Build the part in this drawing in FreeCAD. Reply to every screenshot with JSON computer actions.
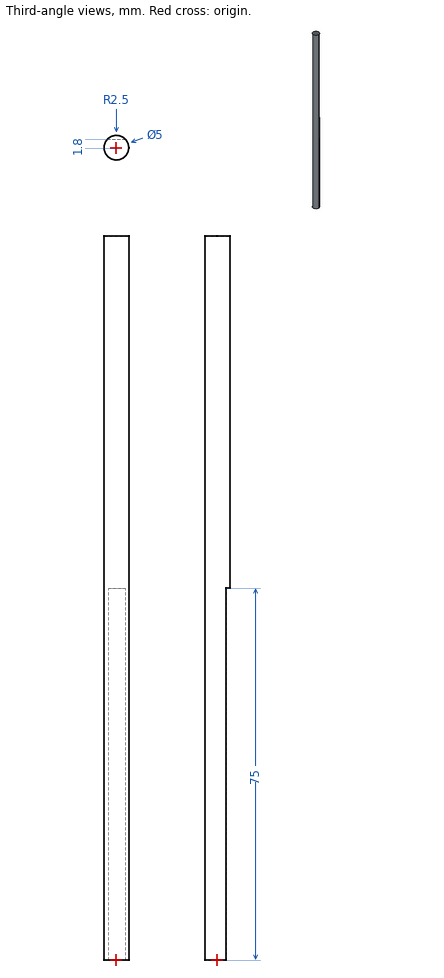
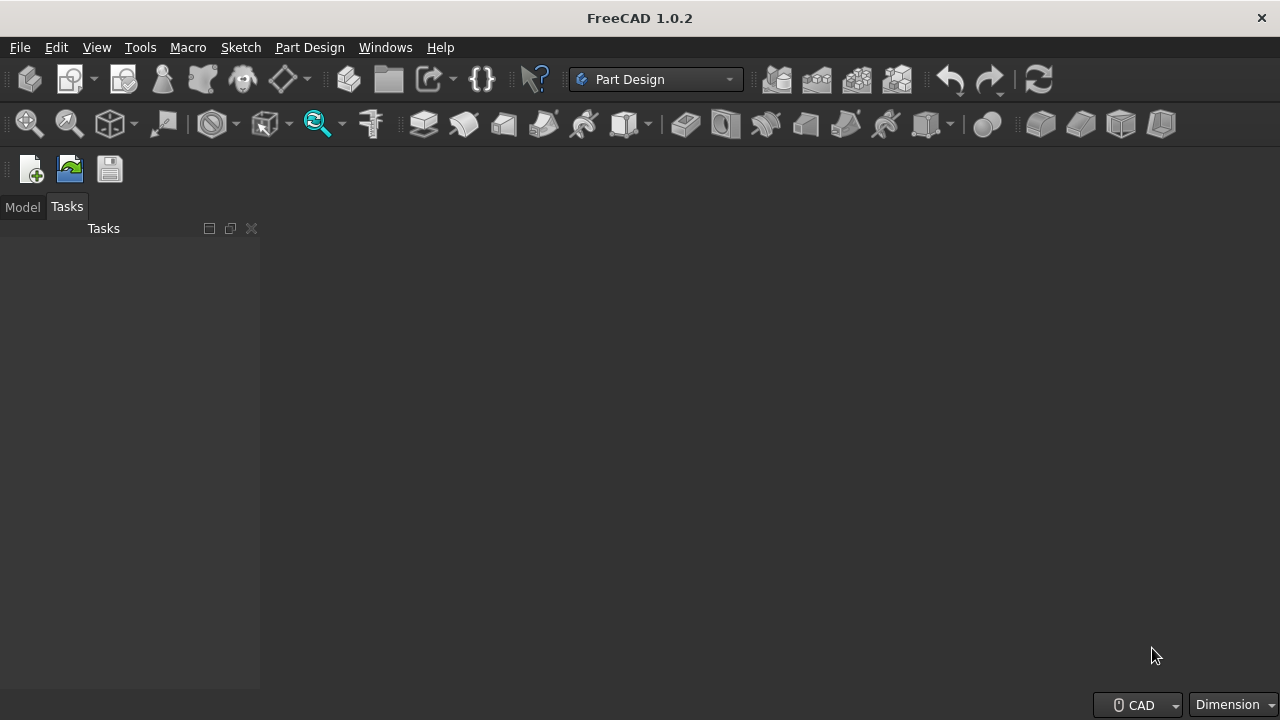
{"action": "key", "text": "ctrl+n"}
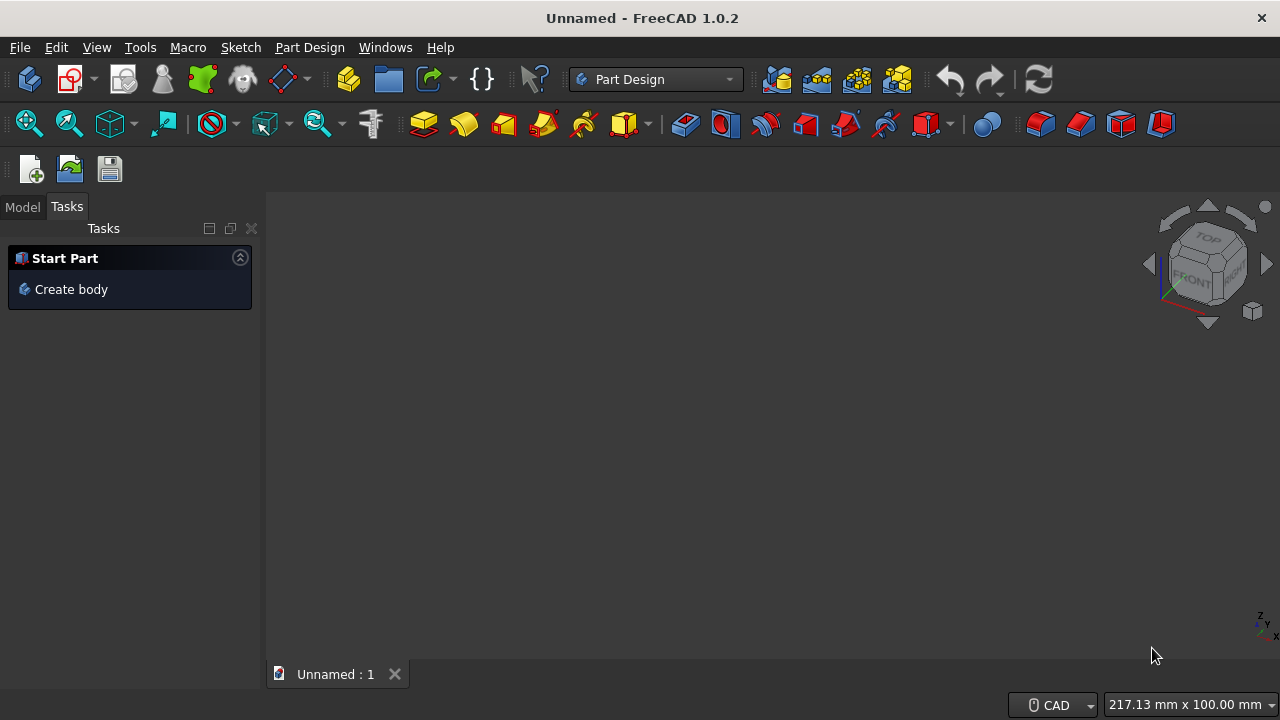
{"action": "left_click", "coordinate": [70, 80]}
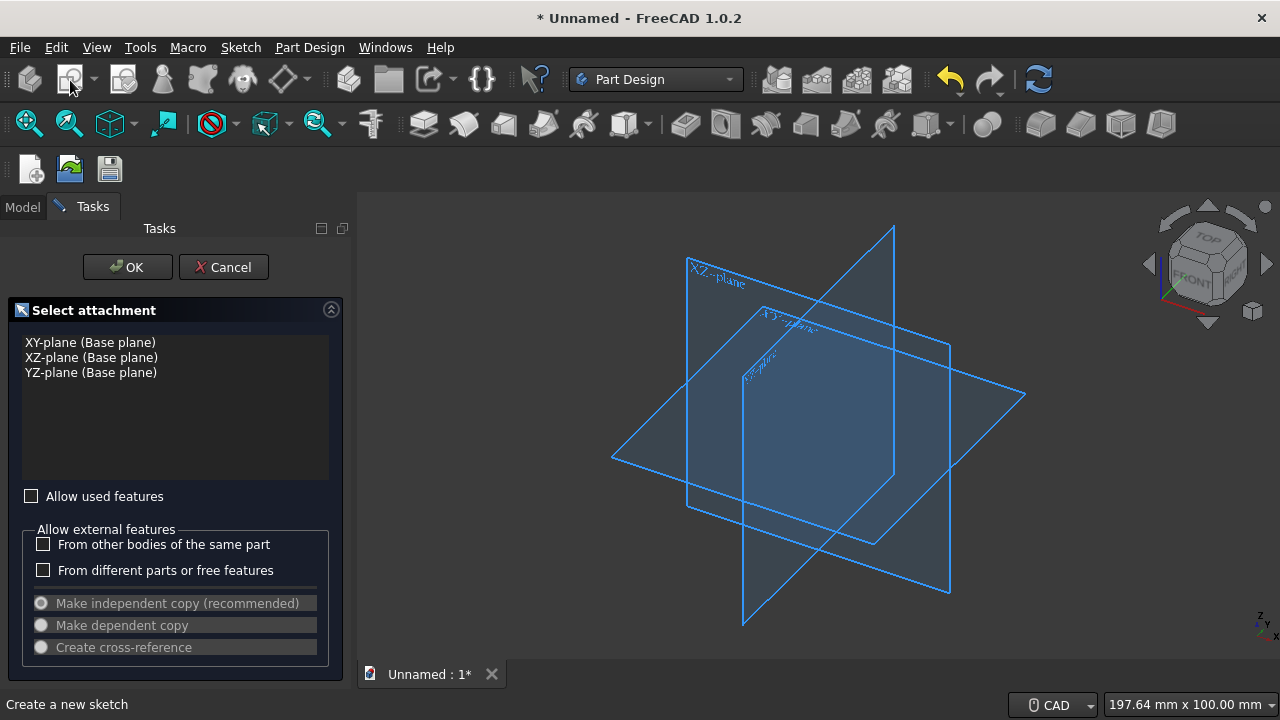
{"action": "left_click", "coordinate": [82, 342]}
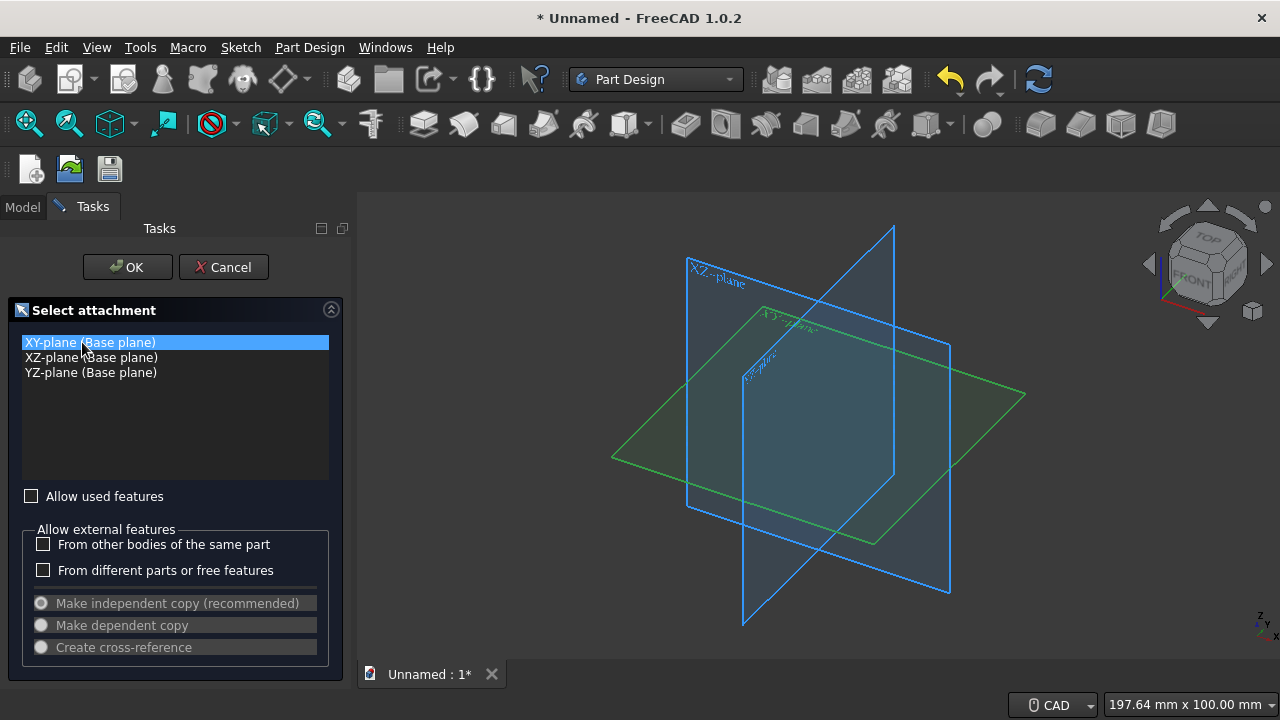
{"action": "left_click", "coordinate": [128, 267]}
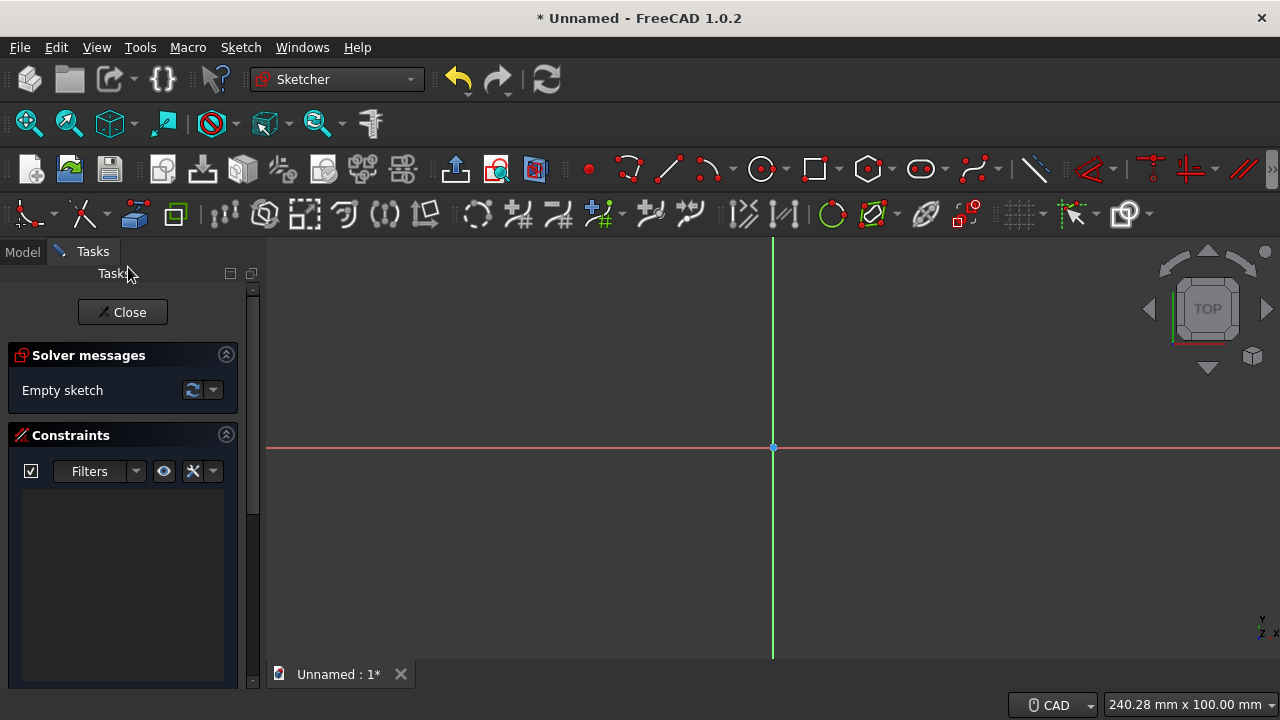
{"action": "scroll", "coordinate": [778, 448], "scroll_direction": "up", "scroll_amount": 13}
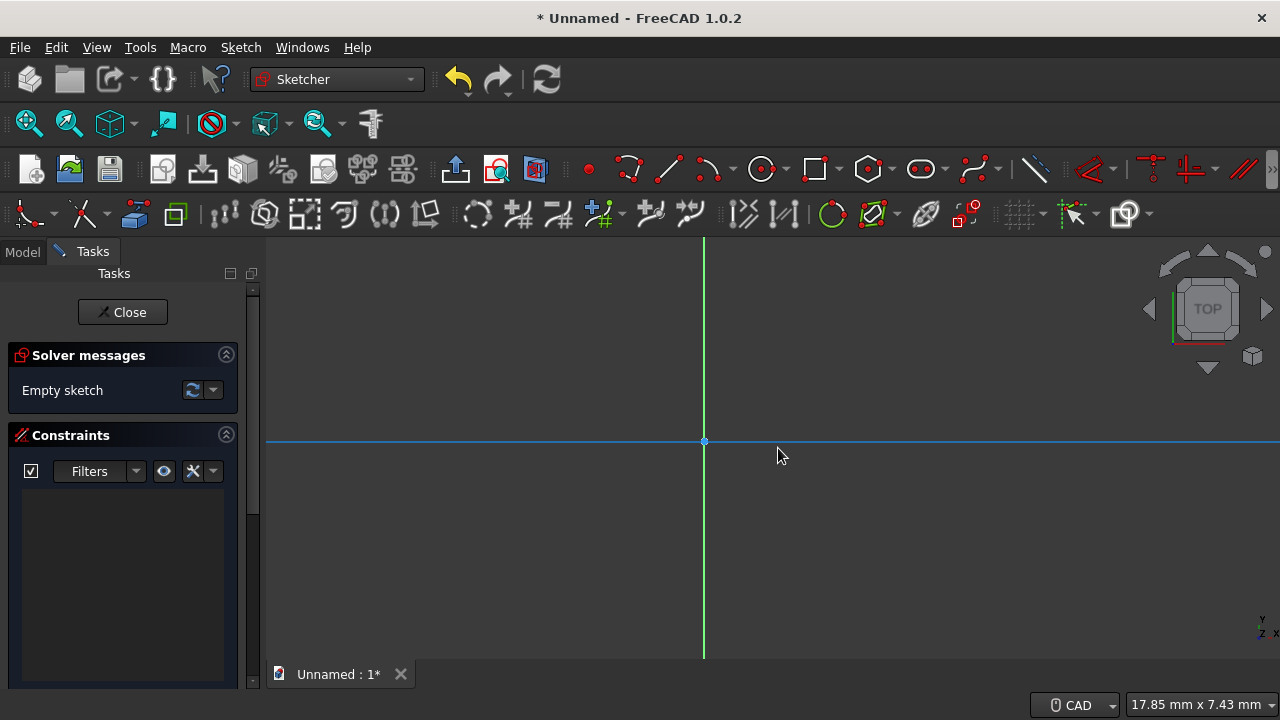
{"action": "key", "text": "g c"}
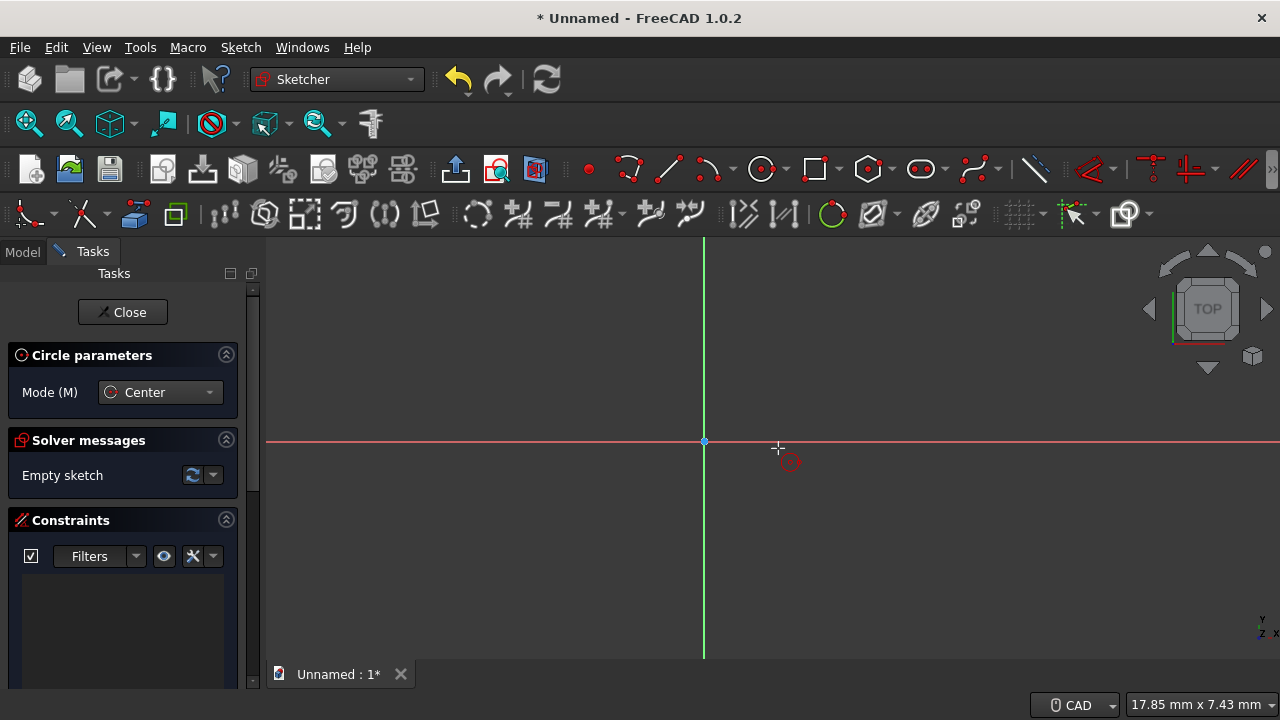
{"action": "left_click", "coordinate": [704, 442]}
{"action": "mouse_move", "coordinate": [805, 341]}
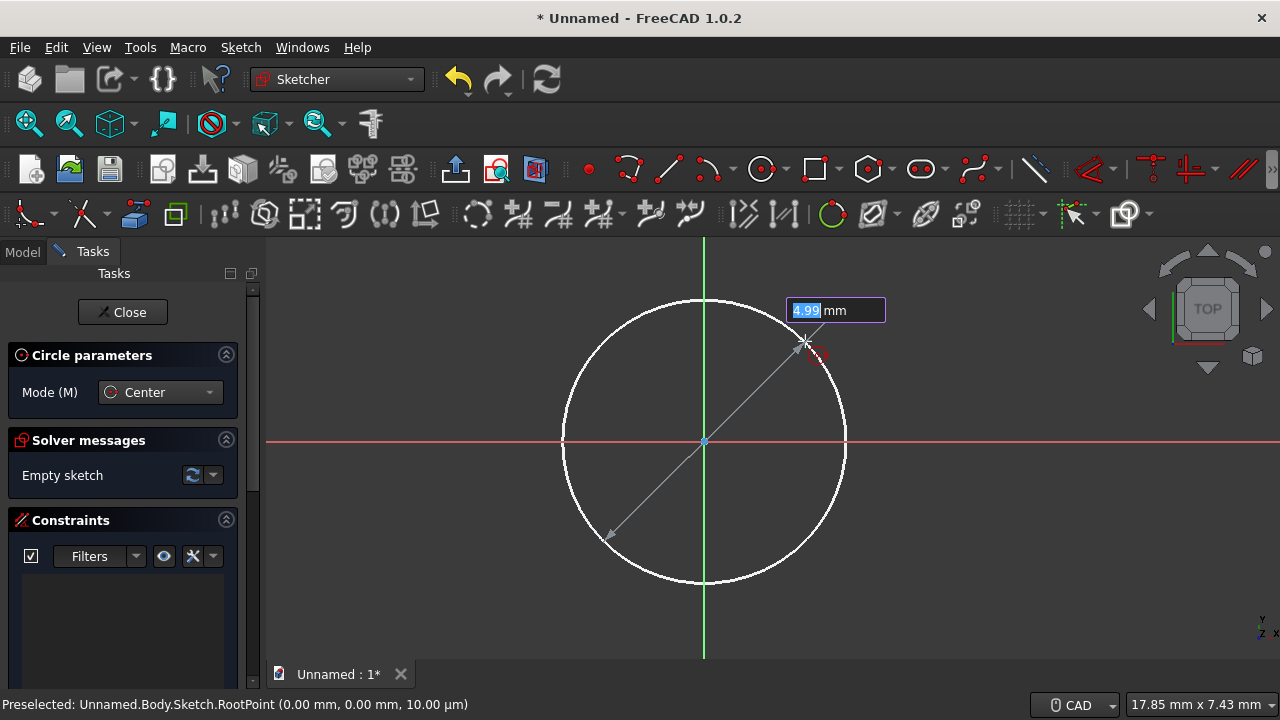
{"action": "type", "text": "5"}
{"action": "key", "text": "Return"}
{"action": "key", "text": "Escape"}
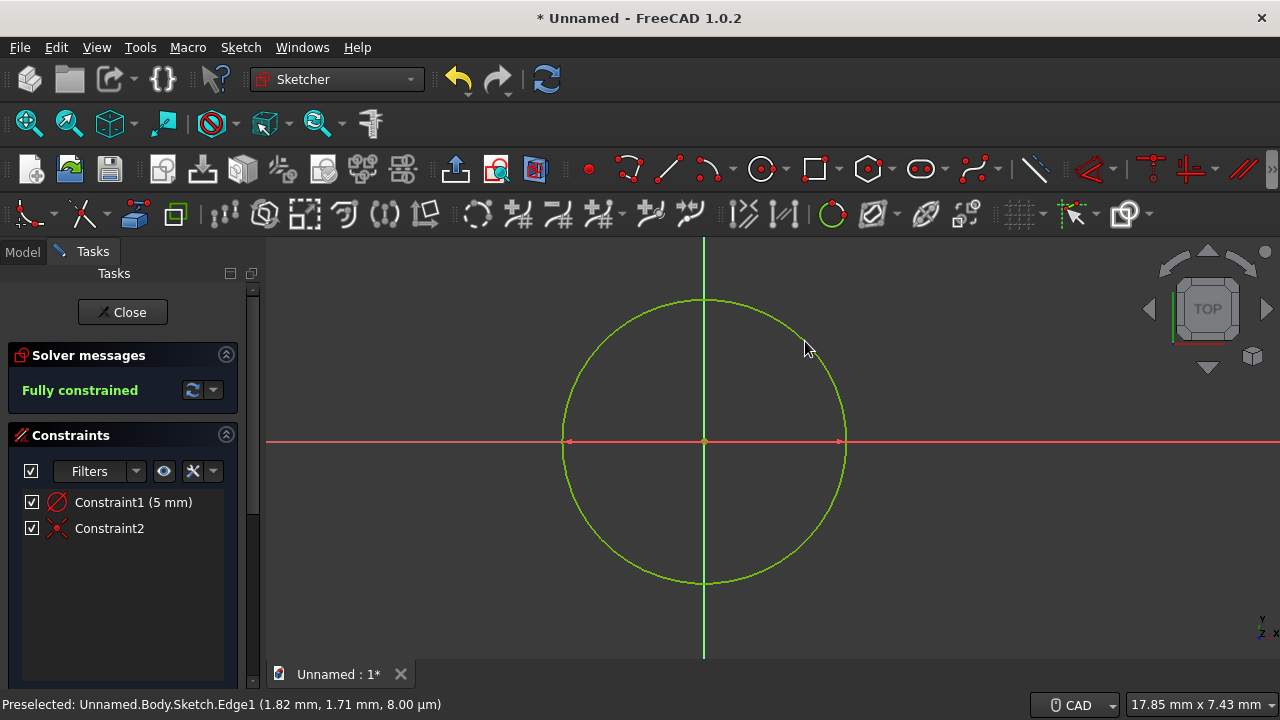
{"action": "left_click", "coordinate": [123, 312]}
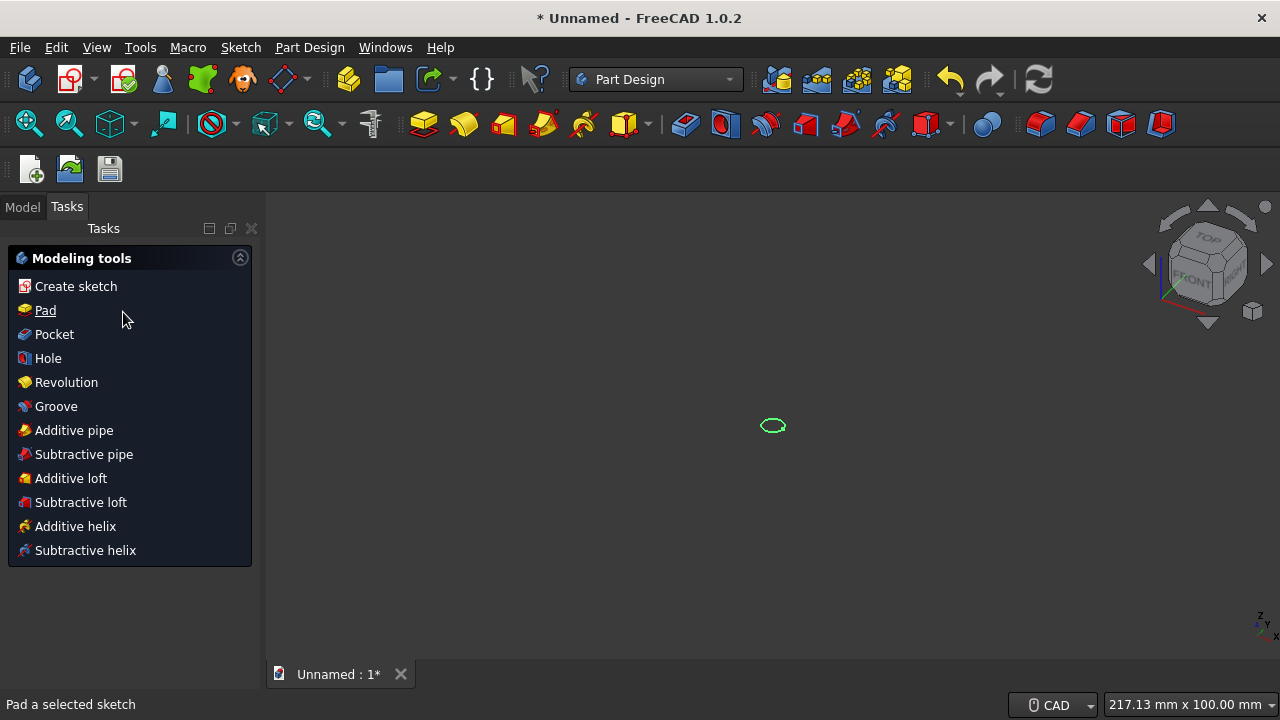
{"action": "left_click", "coordinate": [424, 124]}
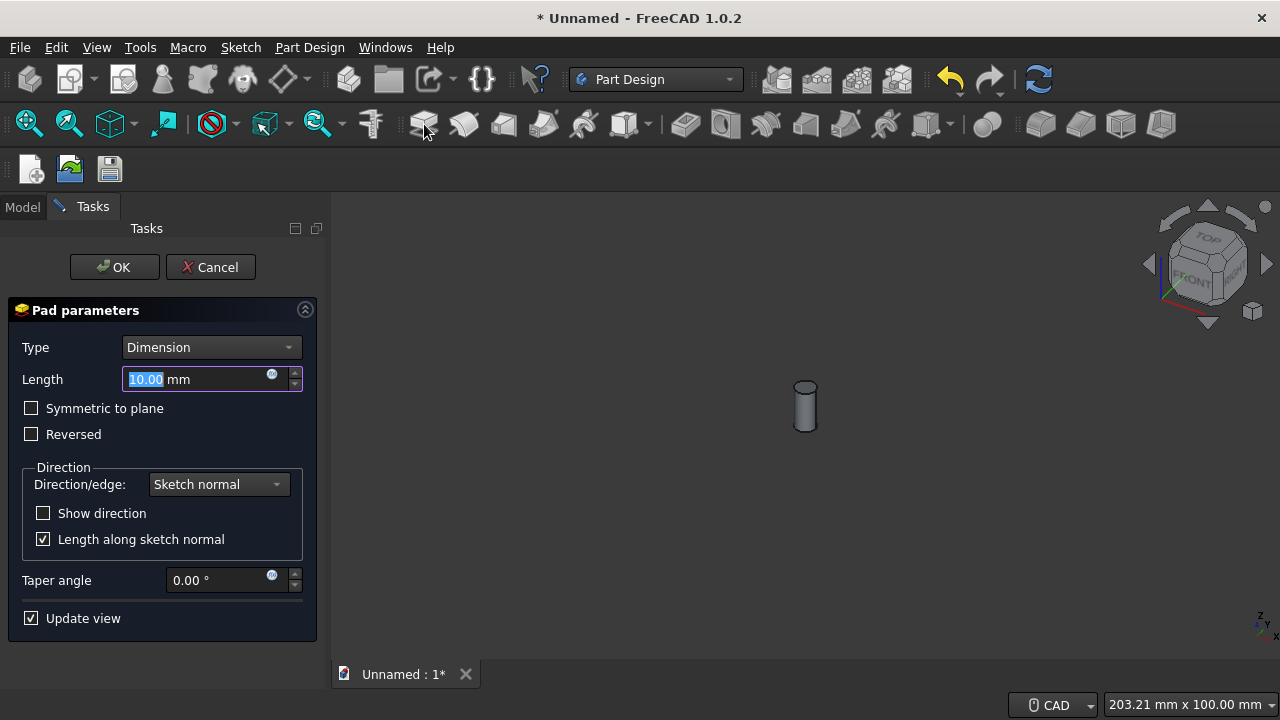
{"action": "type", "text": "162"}
{"action": "key", "text": "Tab"}